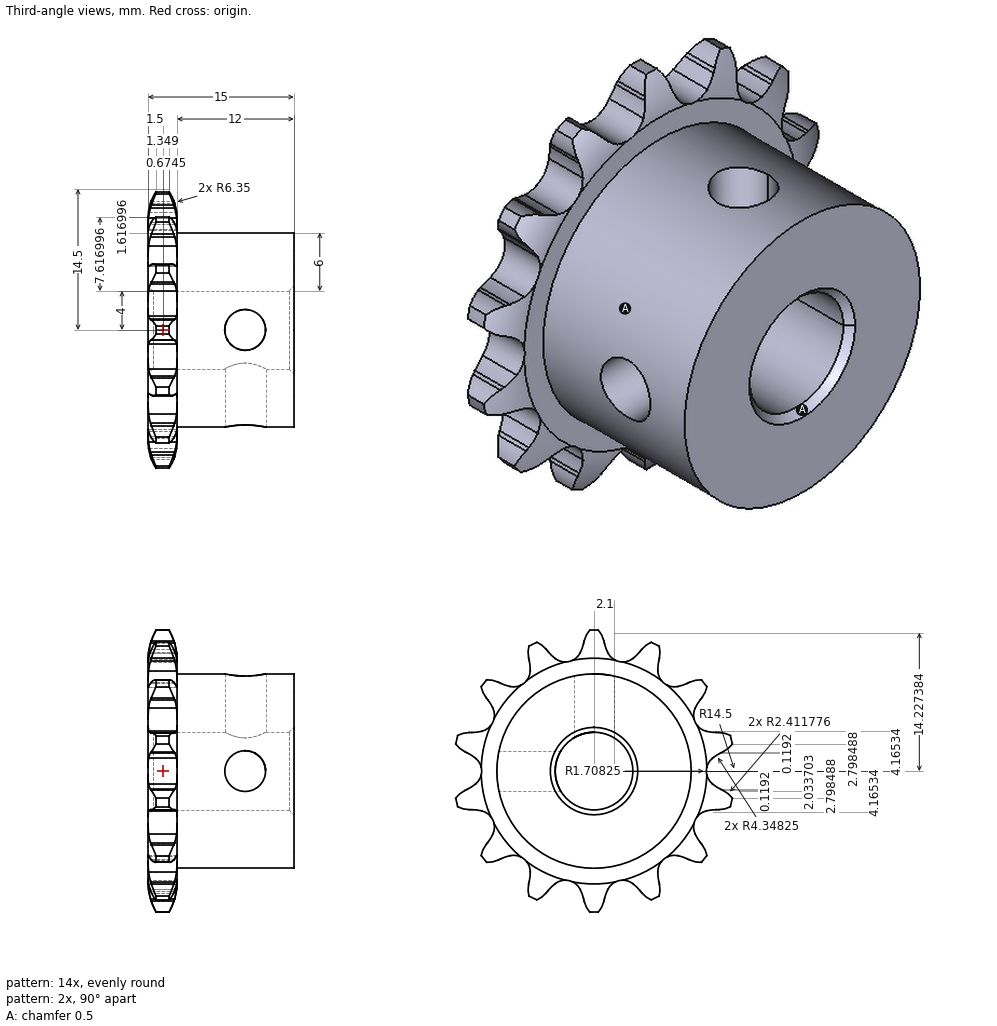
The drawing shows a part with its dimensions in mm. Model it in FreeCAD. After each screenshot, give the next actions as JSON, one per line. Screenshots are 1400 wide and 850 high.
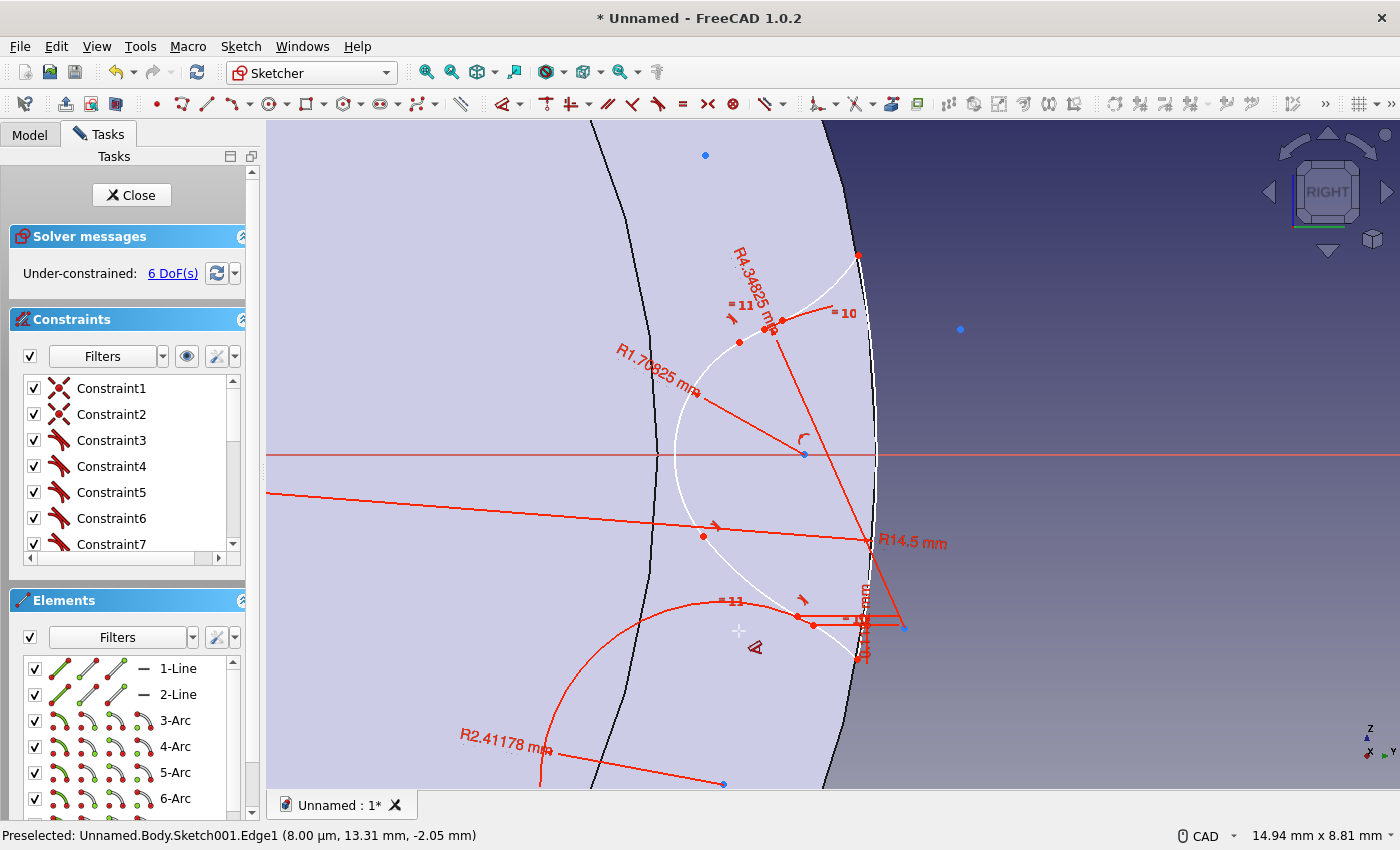
{"action": "scroll", "coordinate": [777, 323], "scroll_direction": "up", "scroll_amount": 8}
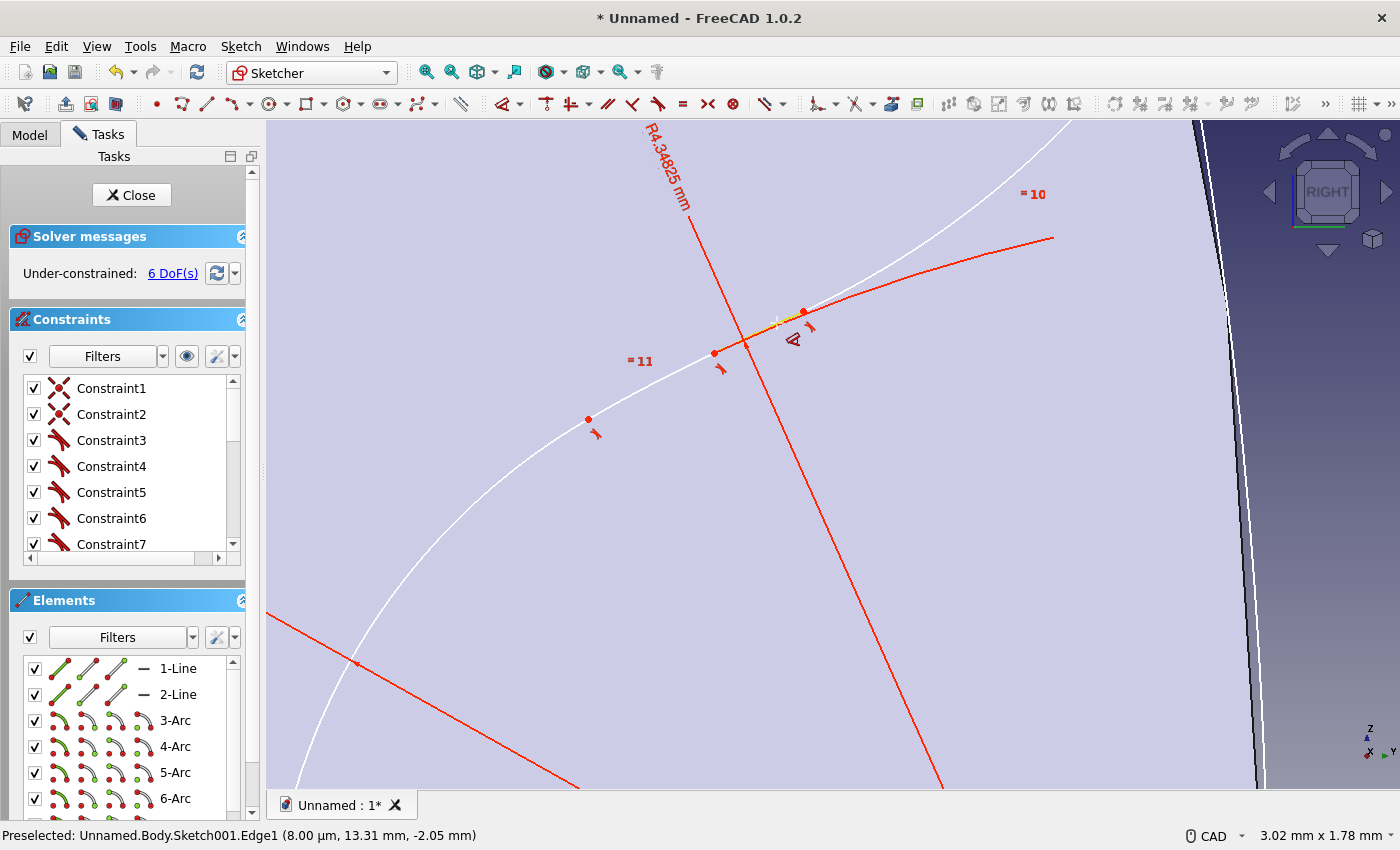
{"action": "left_click", "coordinate": [777, 324]}
{"action": "left_click", "coordinate": [838, 332]}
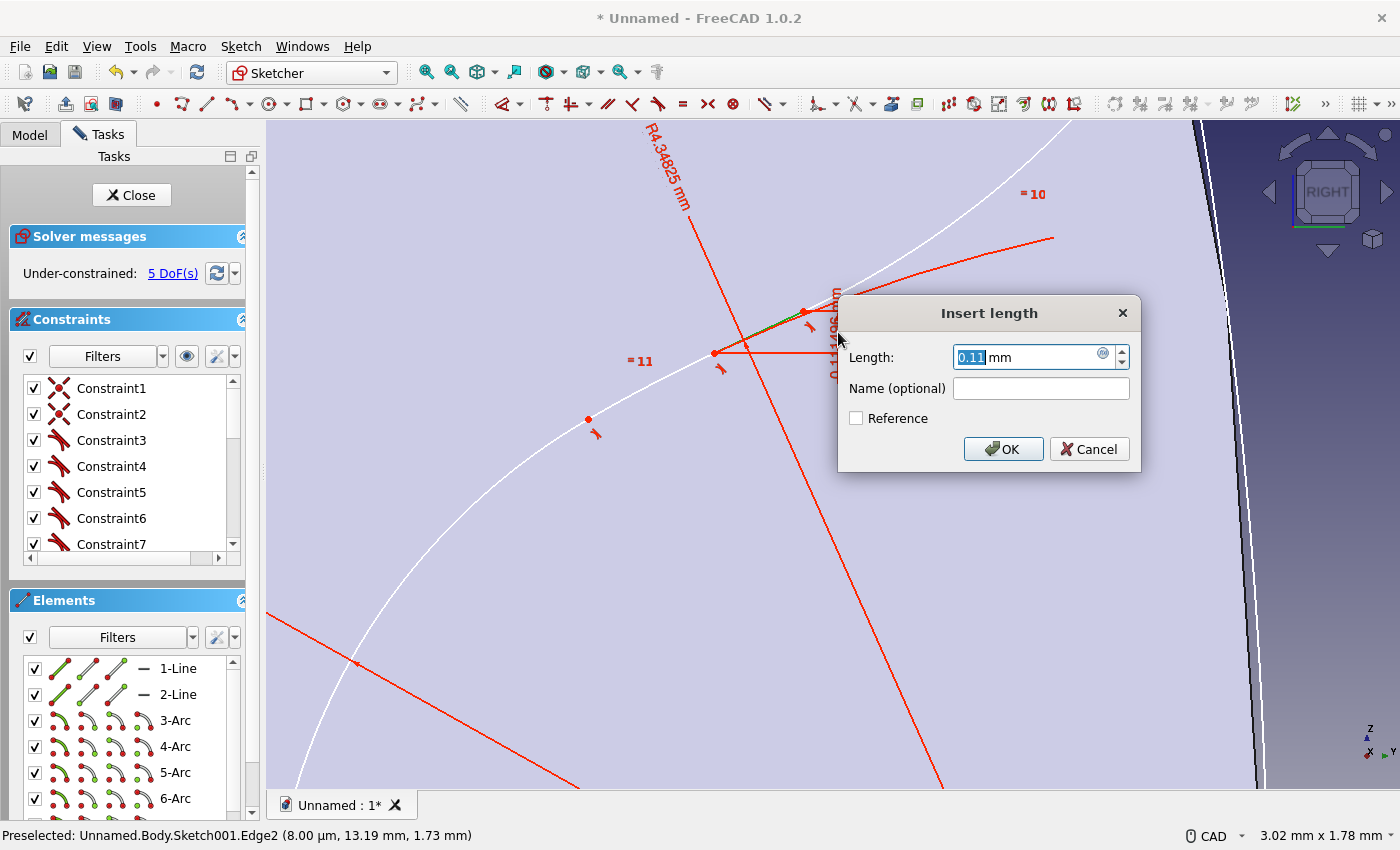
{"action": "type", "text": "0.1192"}
{"action": "key", "text": "Return"}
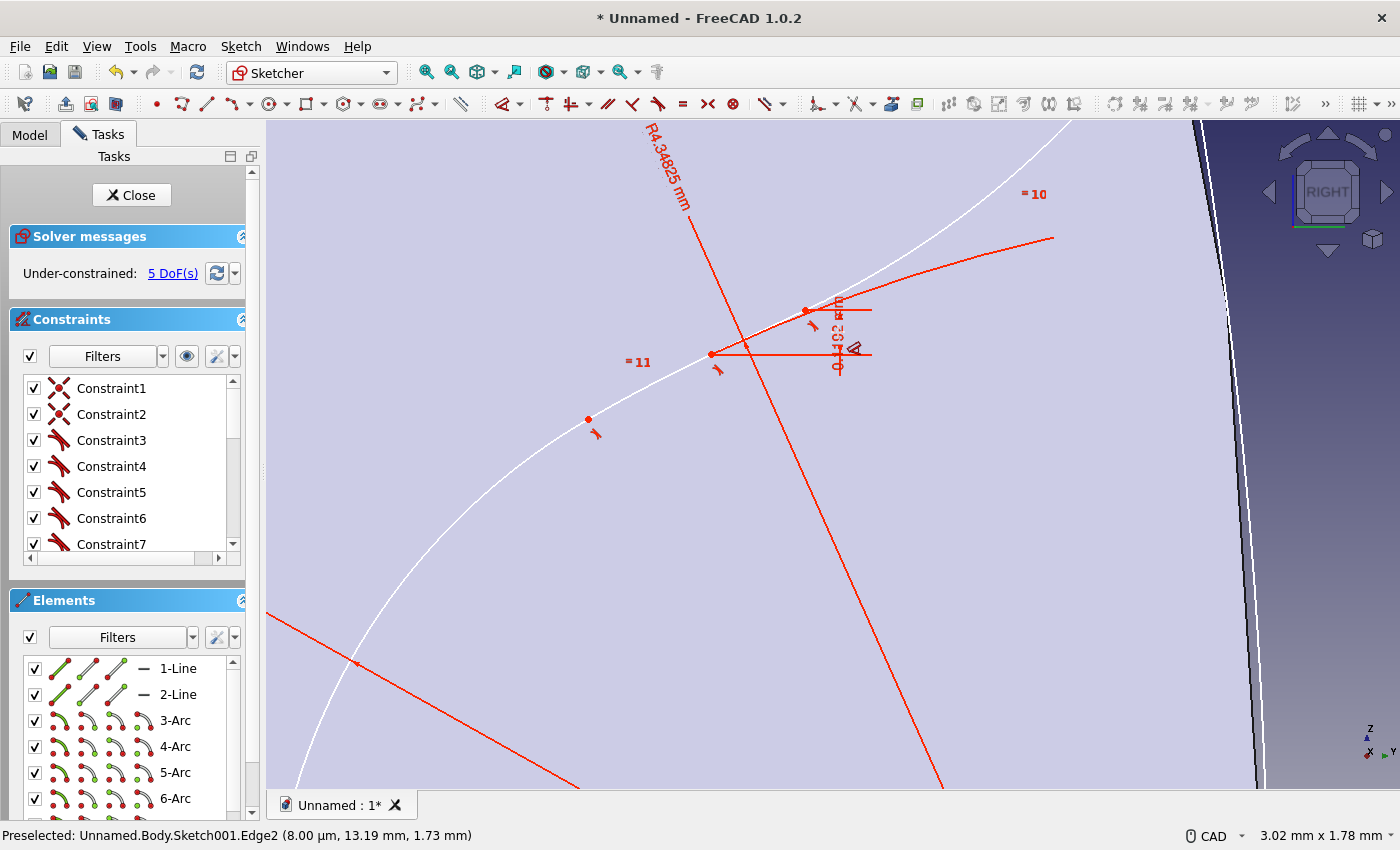
{"action": "scroll", "coordinate": [777, 323], "scroll_direction": "down", "scroll_amount": 8}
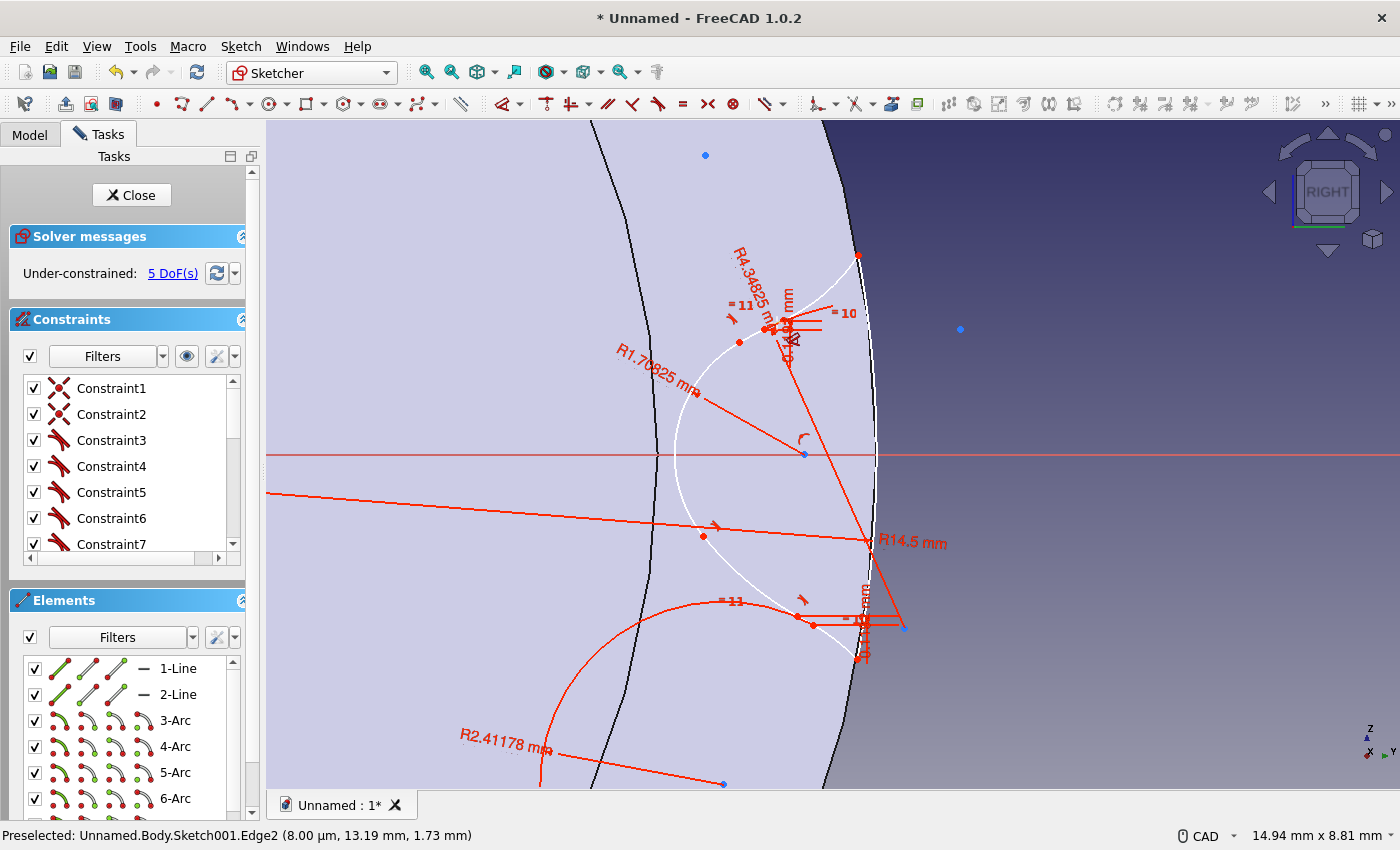
{"action": "scroll", "coordinate": [763, 188], "scroll_direction": "down", "scroll_amount": 1}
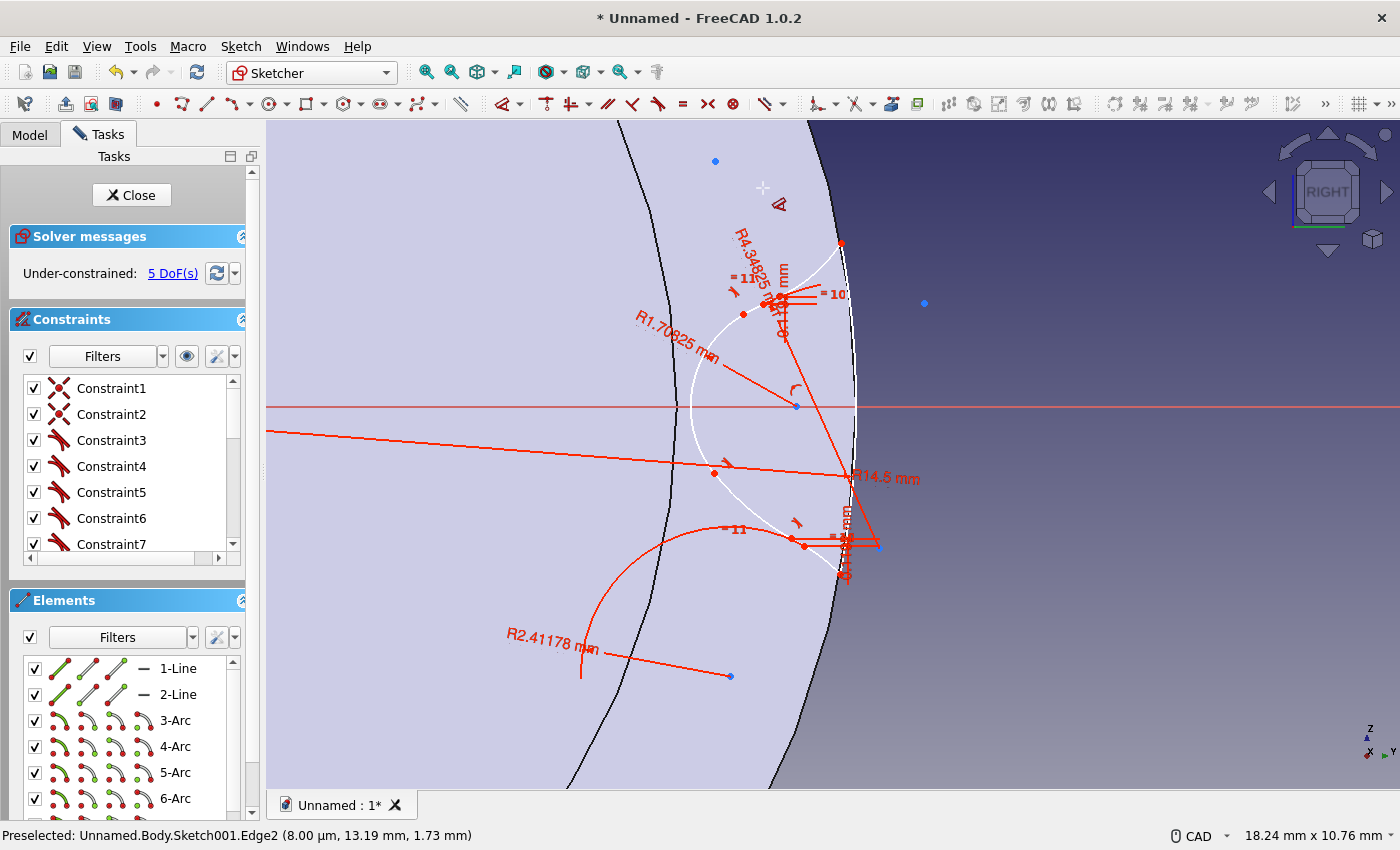
{"action": "left_click", "coordinate": [731, 677]}
{"action": "left_click", "coordinate": [765, 479]}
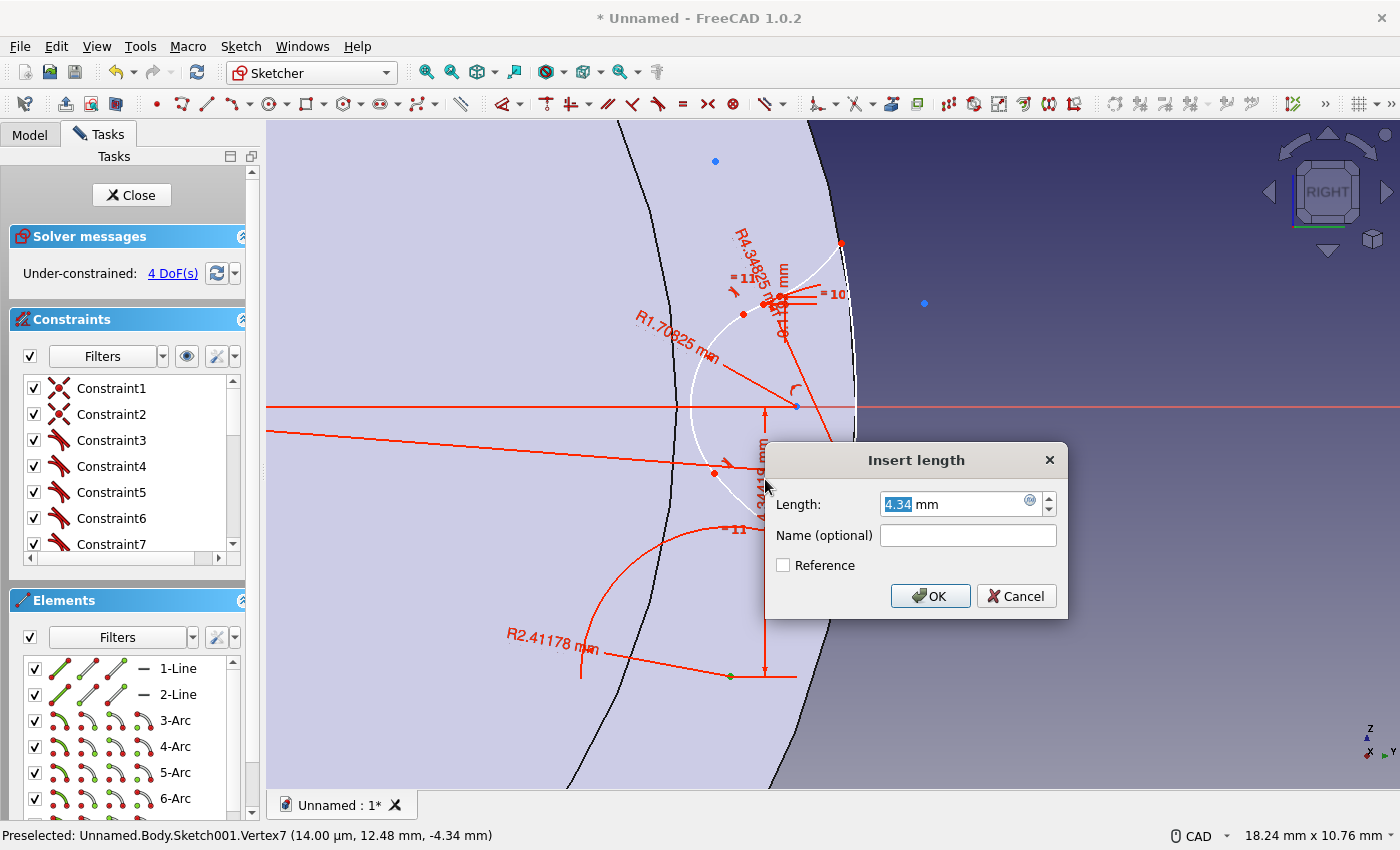
{"action": "type", "text": "4.16534"}
{"action": "key", "text": "Return"}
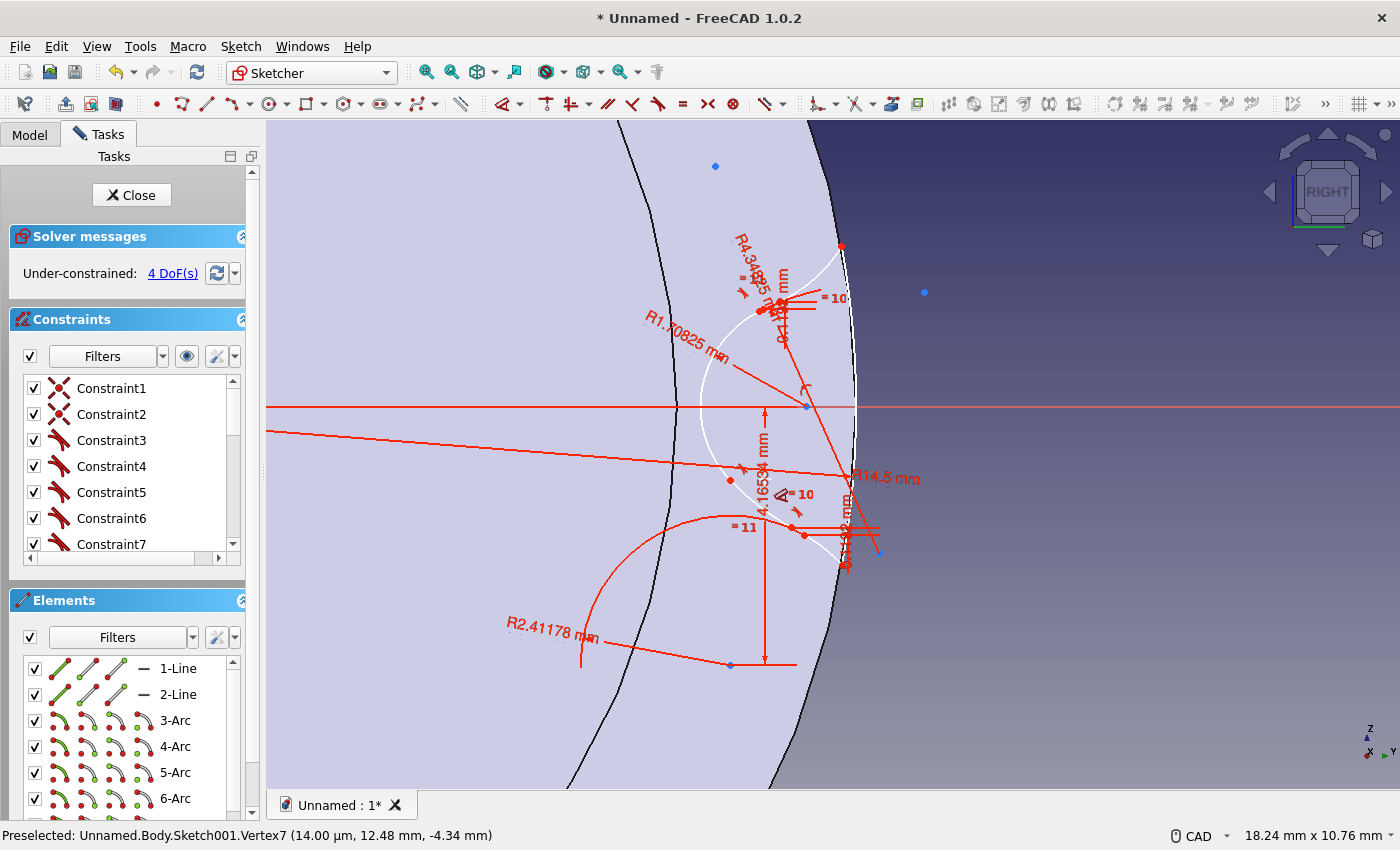
{"action": "left_click", "coordinate": [715, 167]}
{"action": "left_click", "coordinate": [749, 231]}